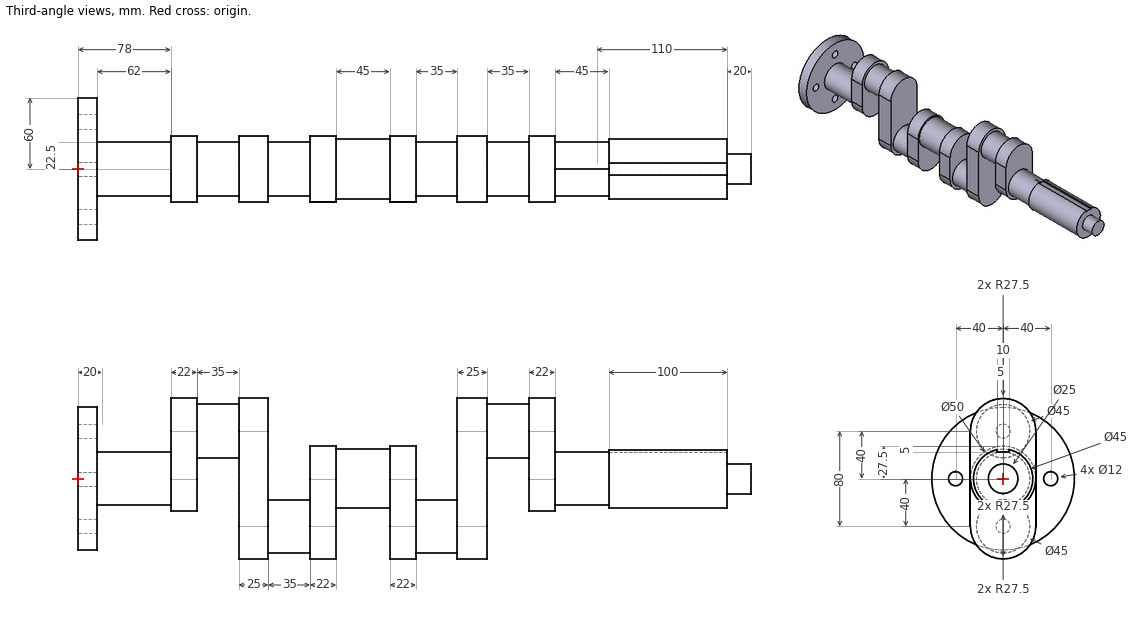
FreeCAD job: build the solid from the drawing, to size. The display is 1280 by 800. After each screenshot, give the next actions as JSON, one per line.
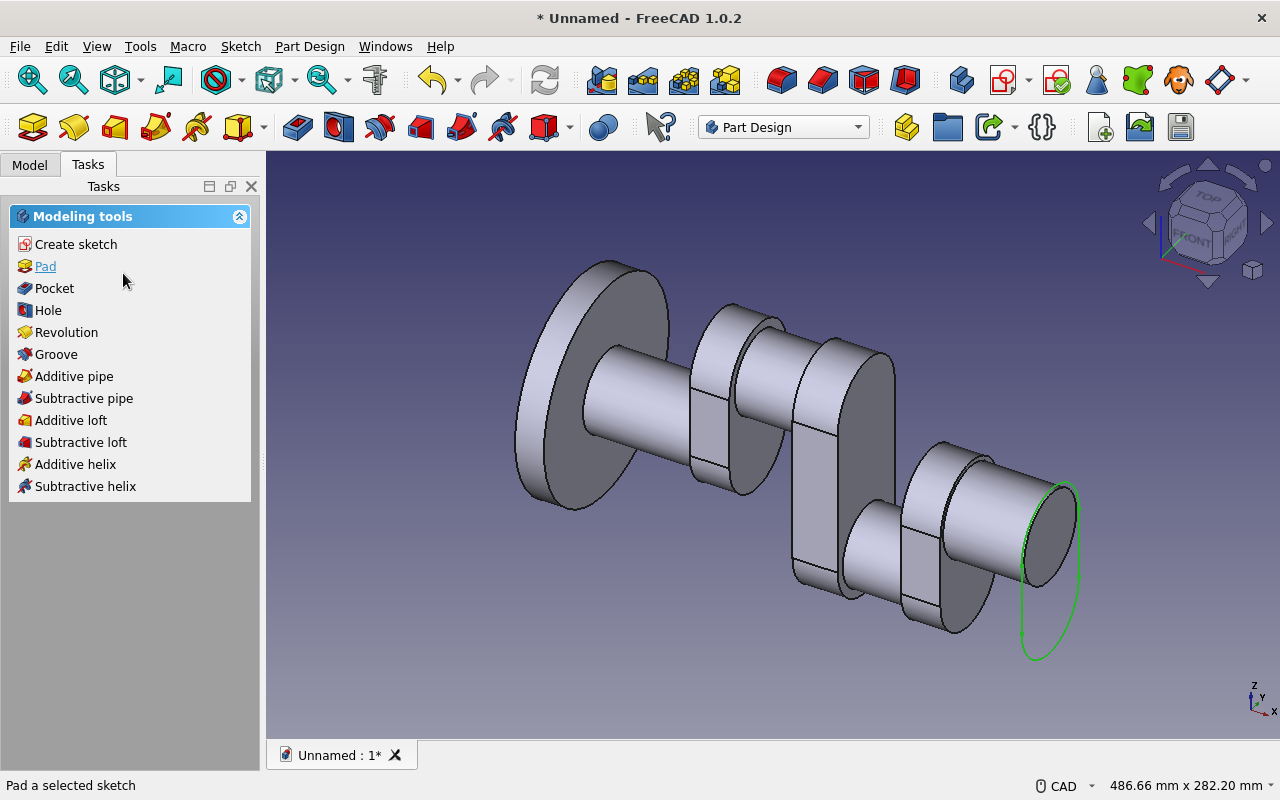
{"action": "left_click", "coordinate": [33, 128]}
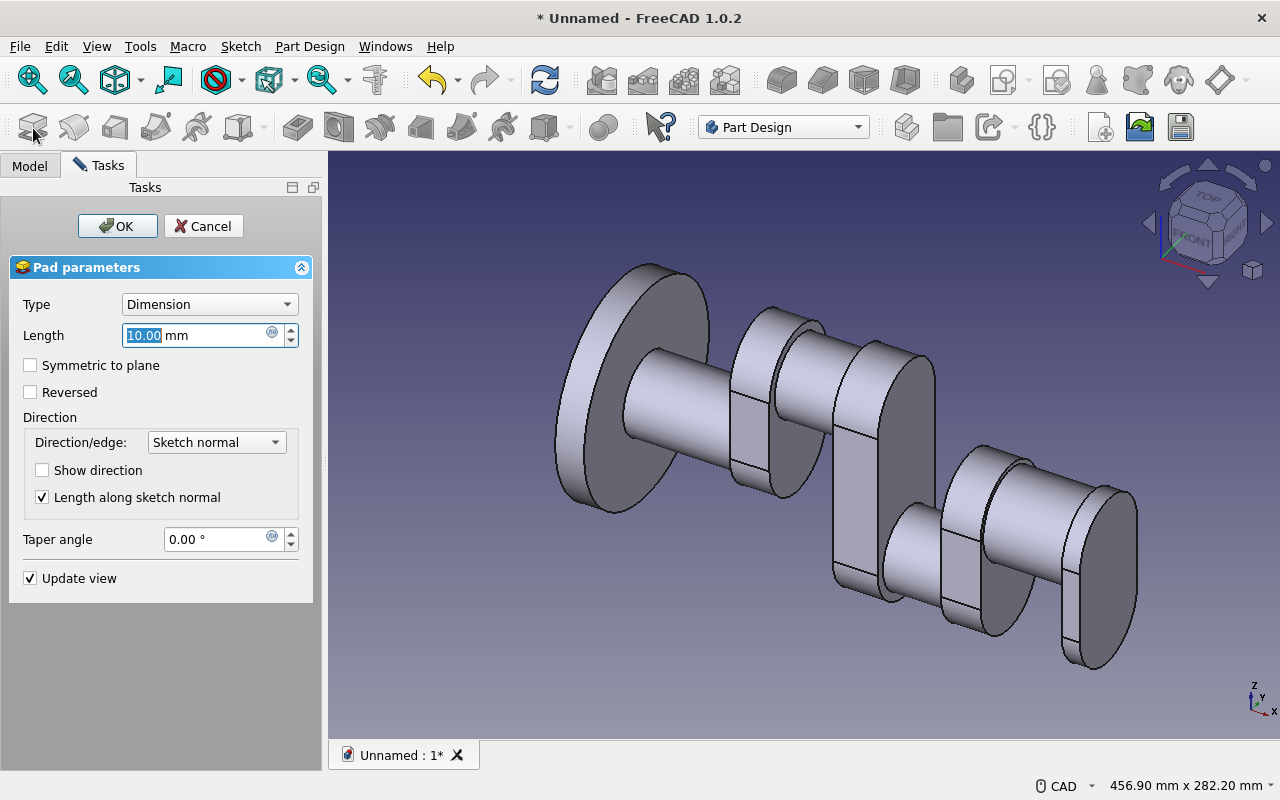
{"action": "type", "text": "22"}
{"action": "key", "text": "Tab"}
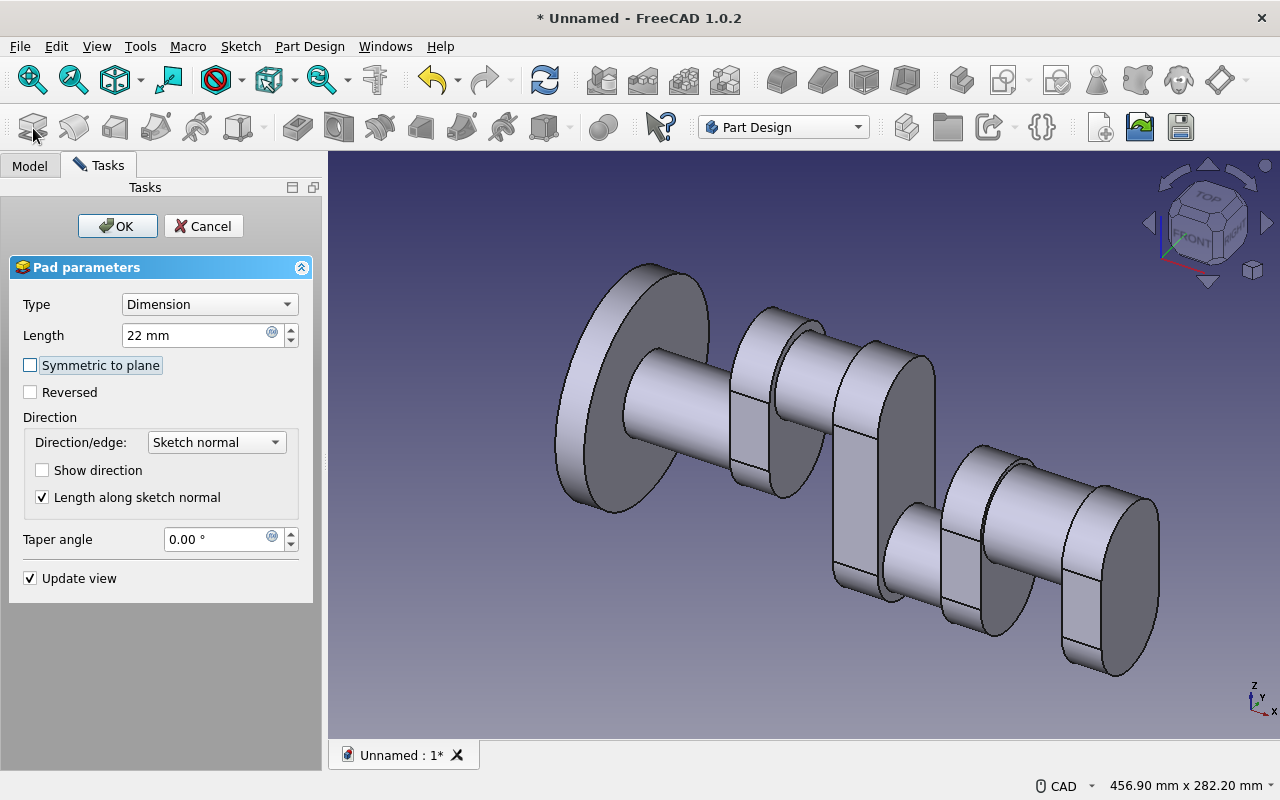
{"action": "left_click", "coordinate": [118, 226]}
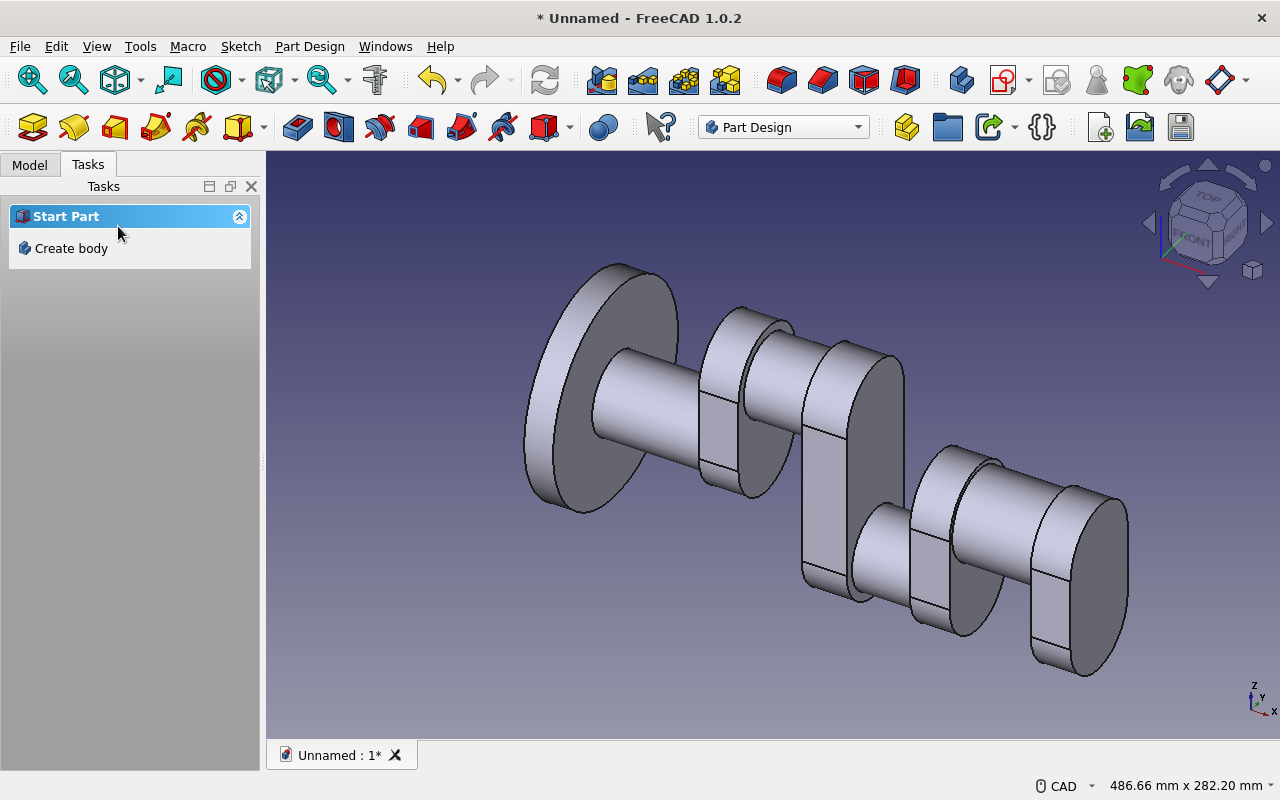
{"action": "left_click", "coordinate": [1099, 563]}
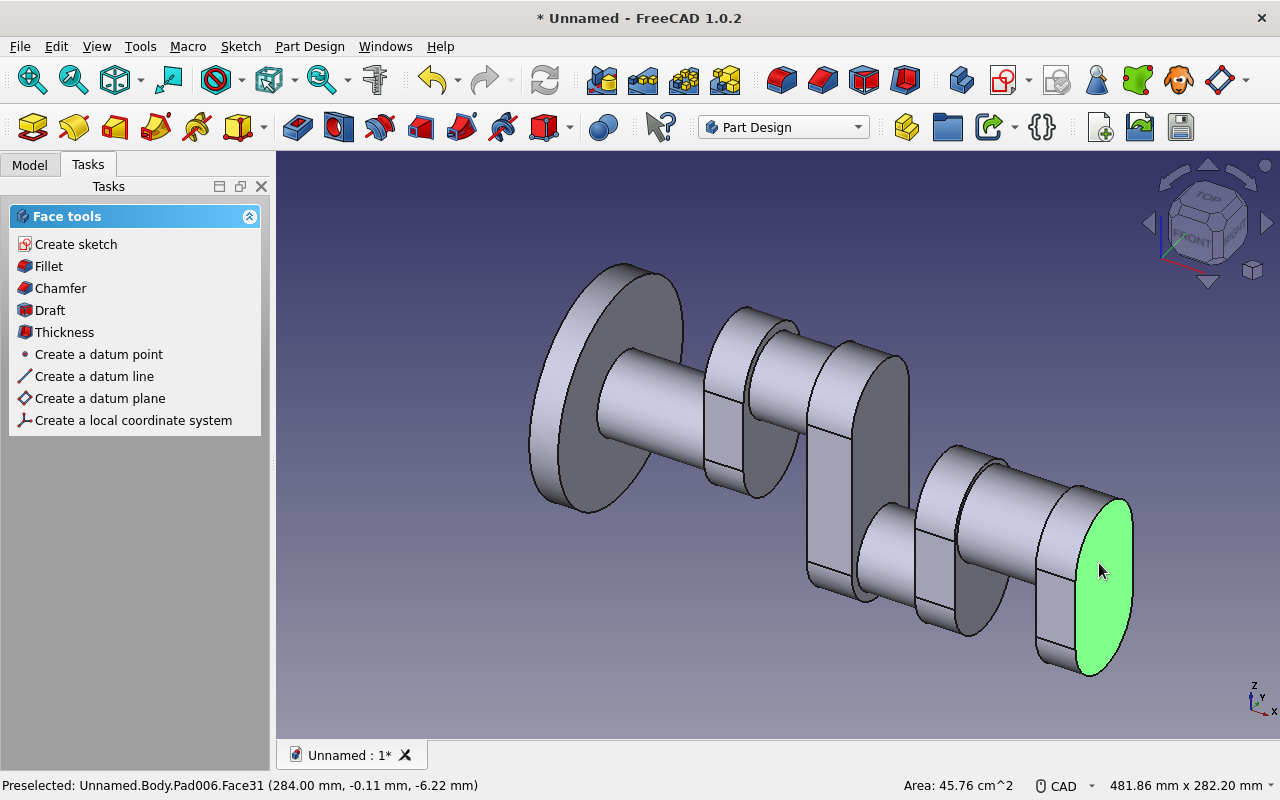
{"action": "left_click", "coordinate": [1002, 80]}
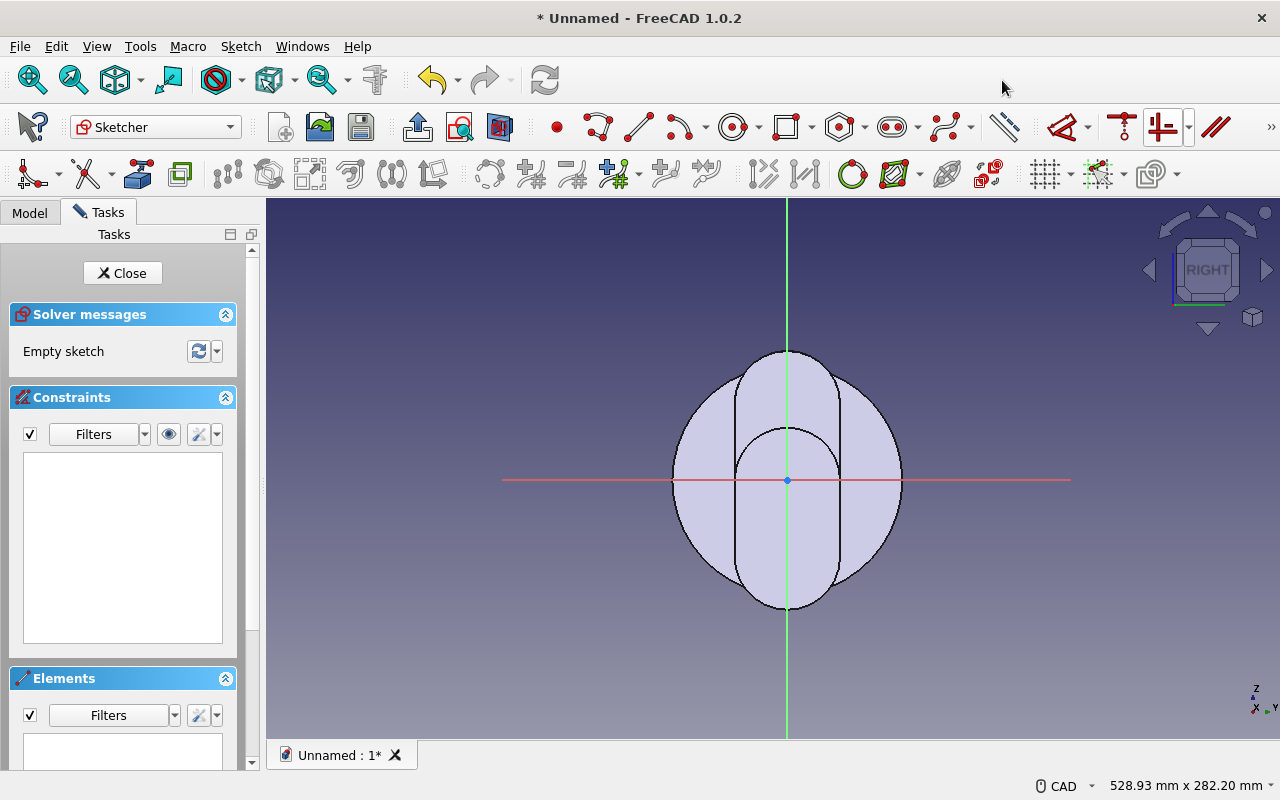
{"action": "scroll", "coordinate": [836, 582], "scroll_direction": "up", "scroll_amount": 5}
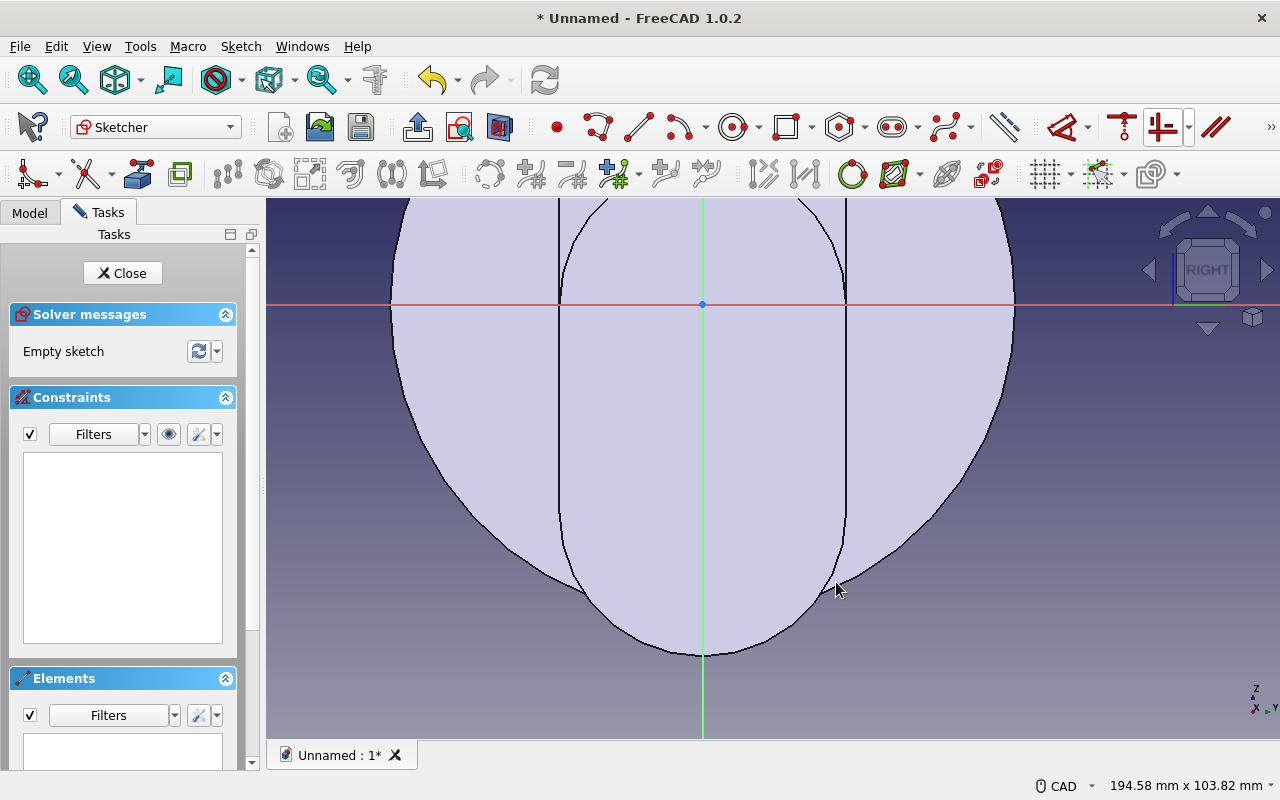
{"action": "key", "text": "g c"}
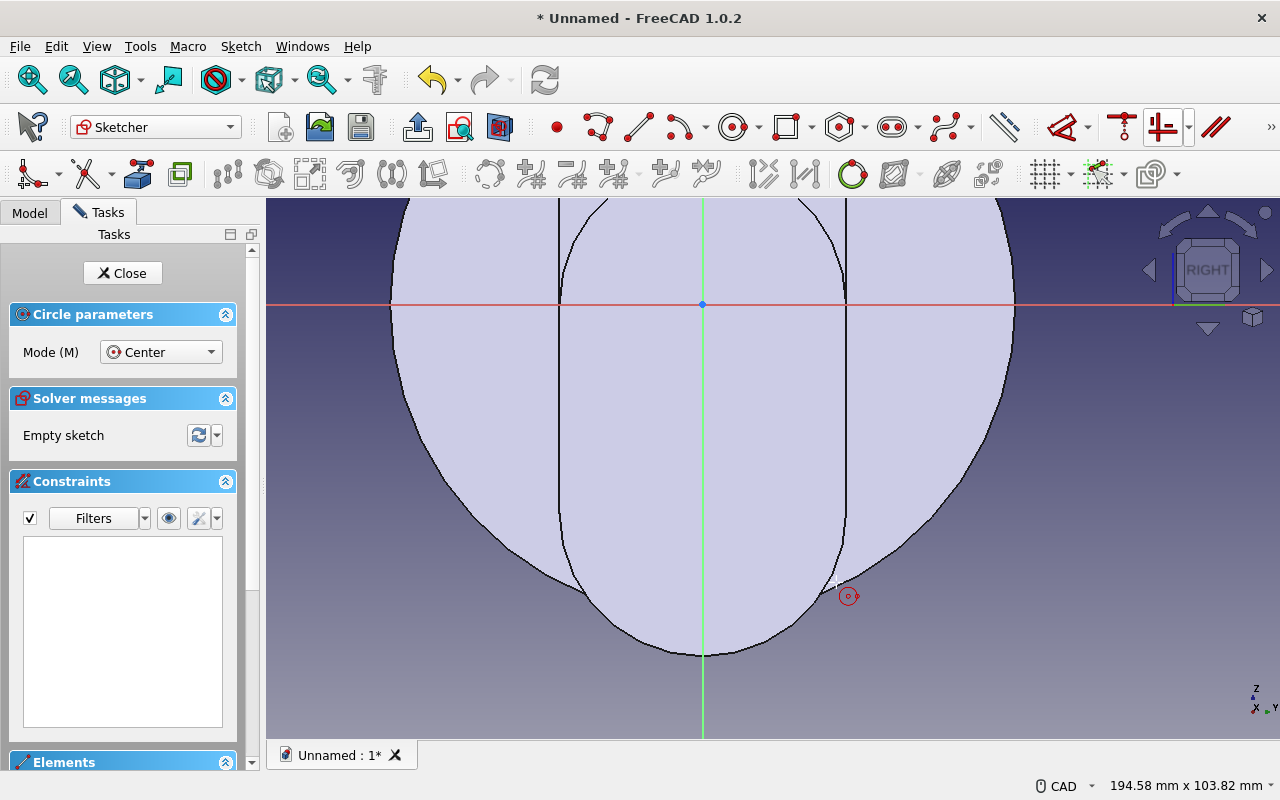
{"action": "left_click", "coordinate": [703, 513]}
{"action": "left_click", "coordinate": [786, 430]}
{"action": "key", "text": "Escape"}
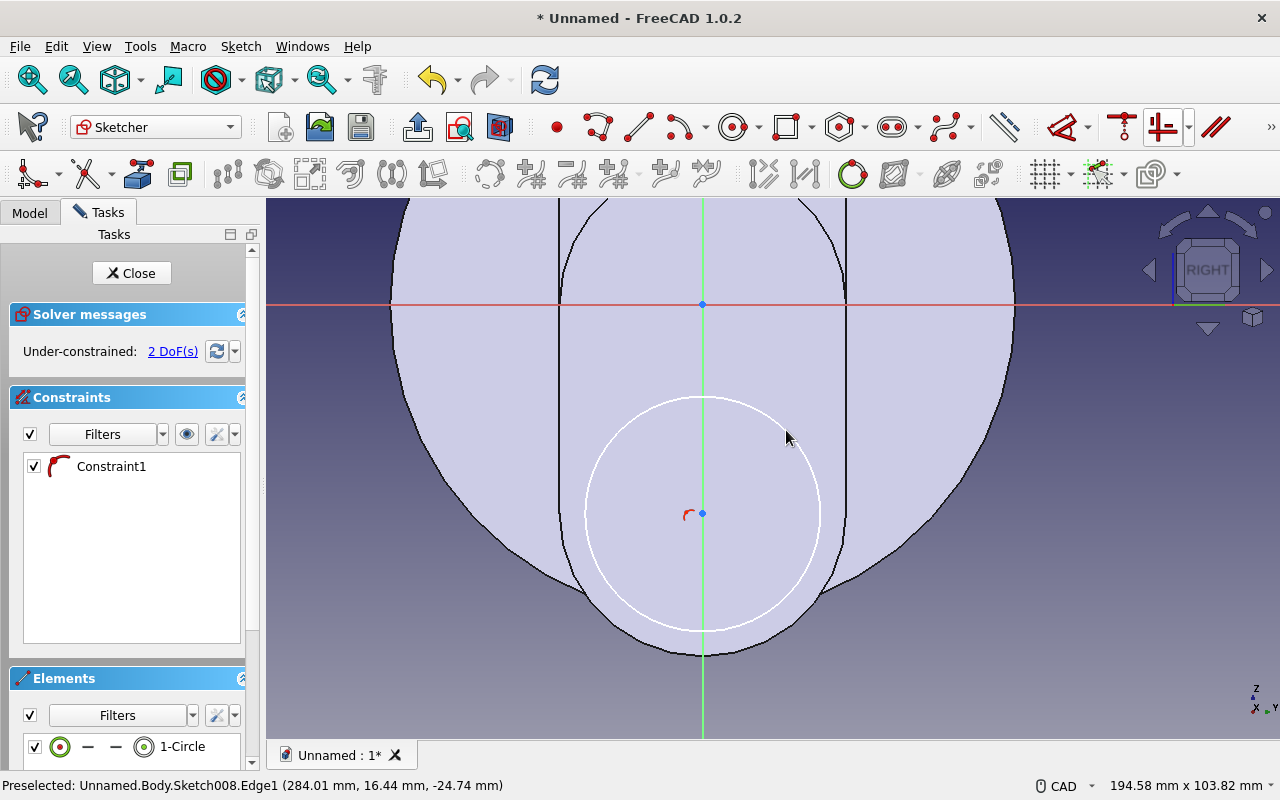
{"action": "left_click", "coordinate": [1062, 128]}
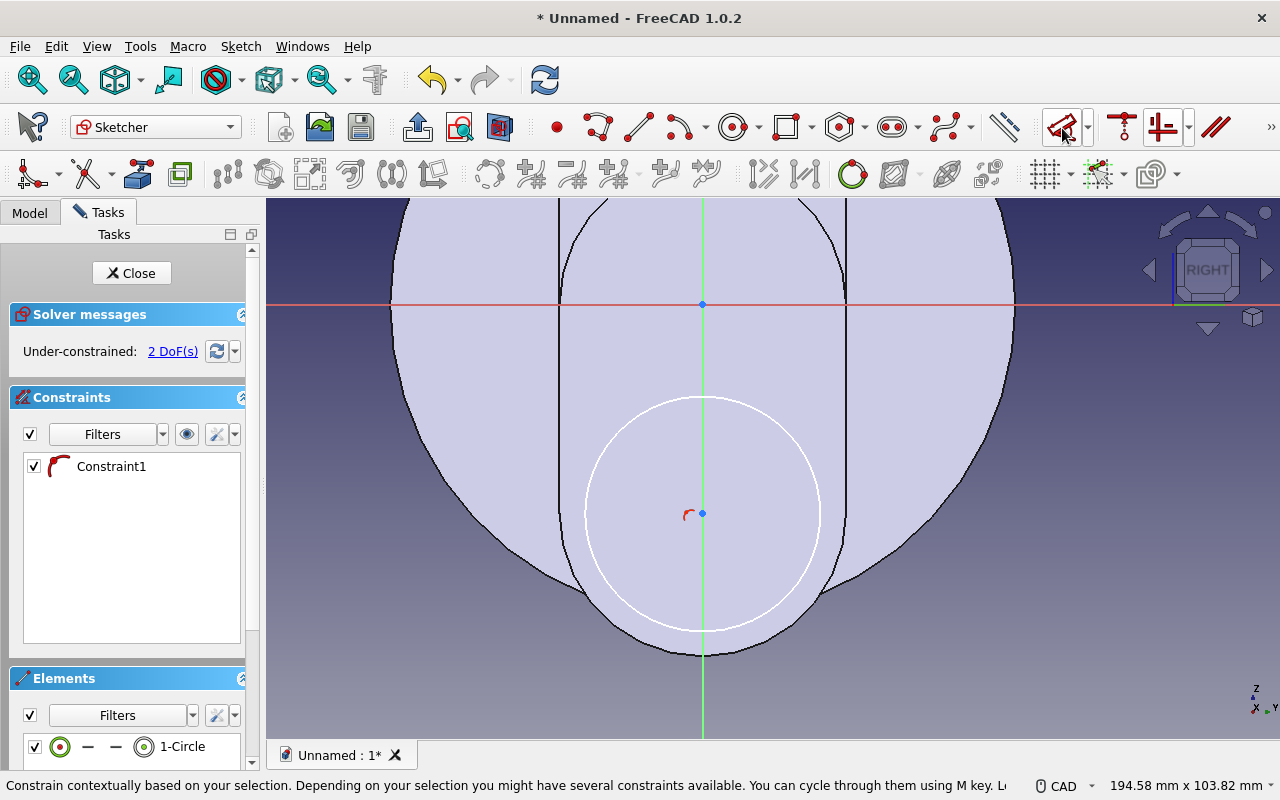
{"action": "left_click", "coordinate": [786, 431]}
{"action": "left_click", "coordinate": [809, 408]}